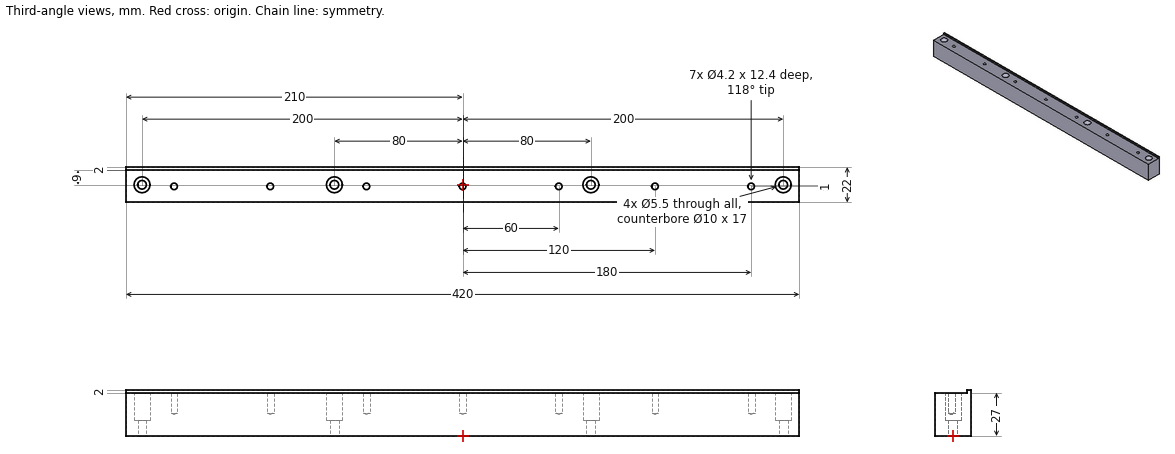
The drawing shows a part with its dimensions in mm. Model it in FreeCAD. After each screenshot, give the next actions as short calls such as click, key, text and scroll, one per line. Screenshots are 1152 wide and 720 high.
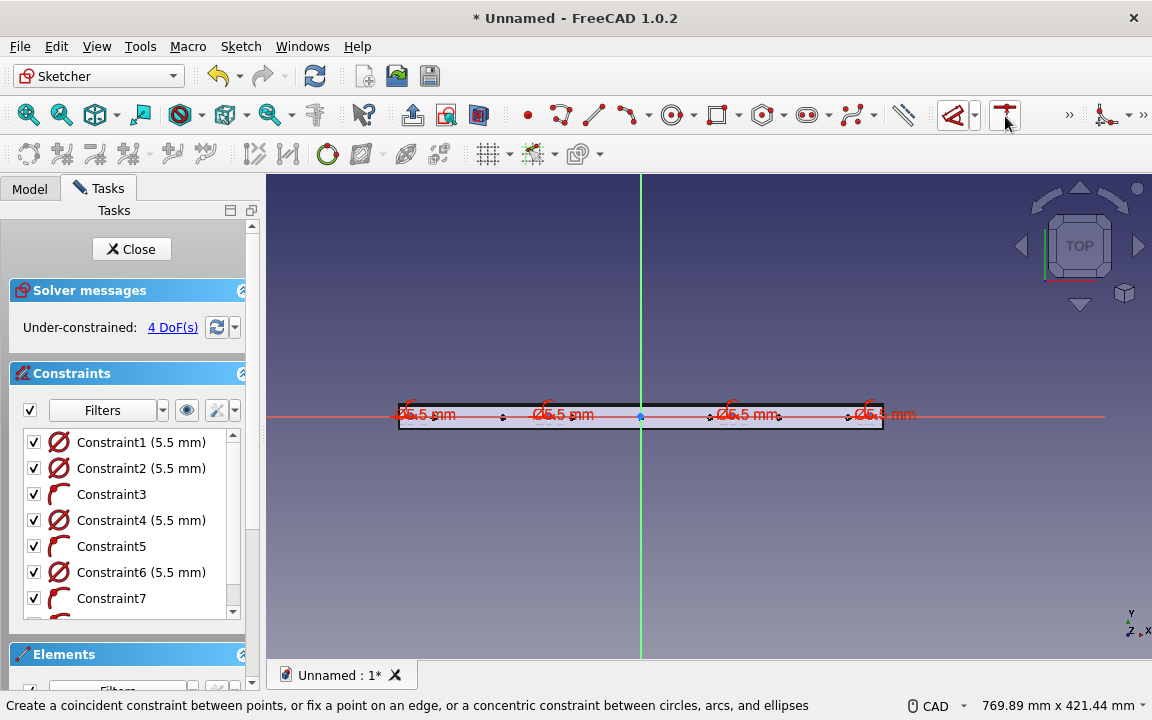
click(733, 417)
click(687, 451)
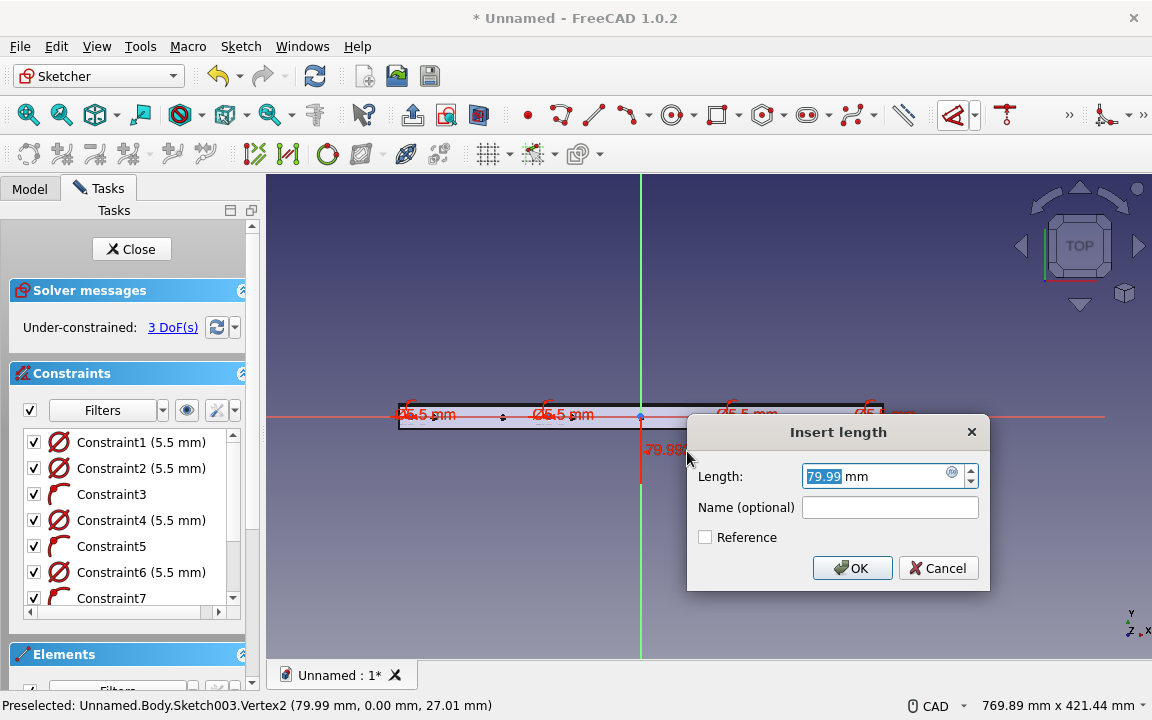
text(80)
key(Return)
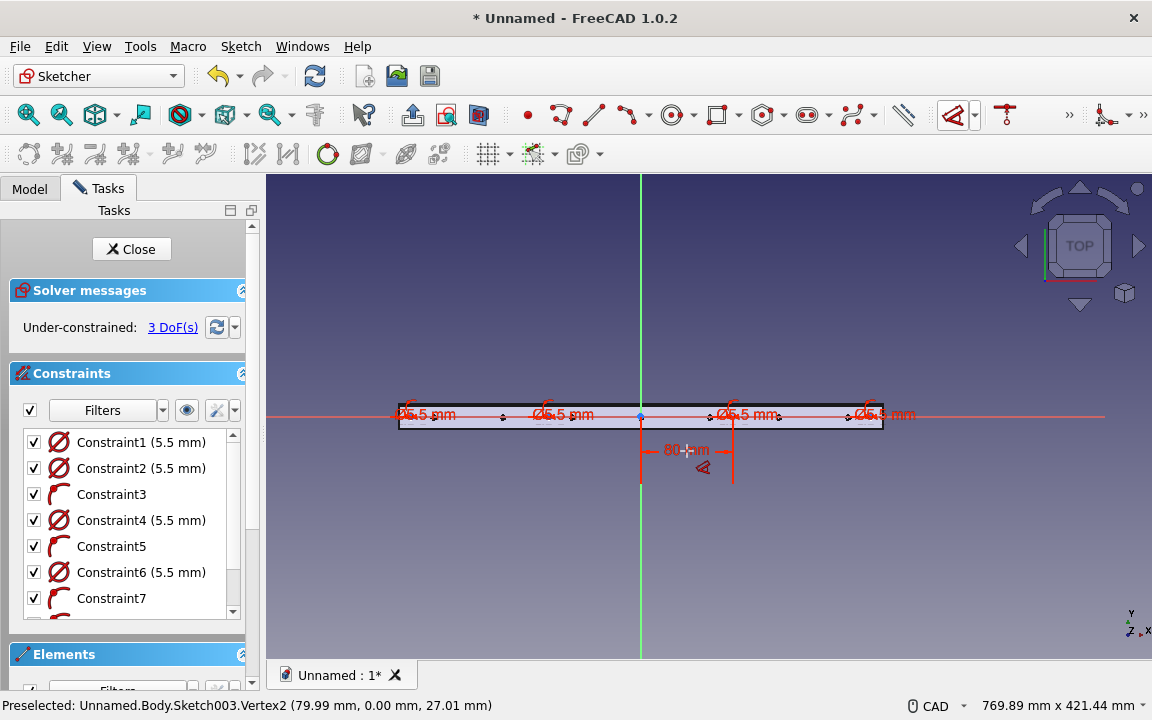
click(549, 417)
click(595, 451)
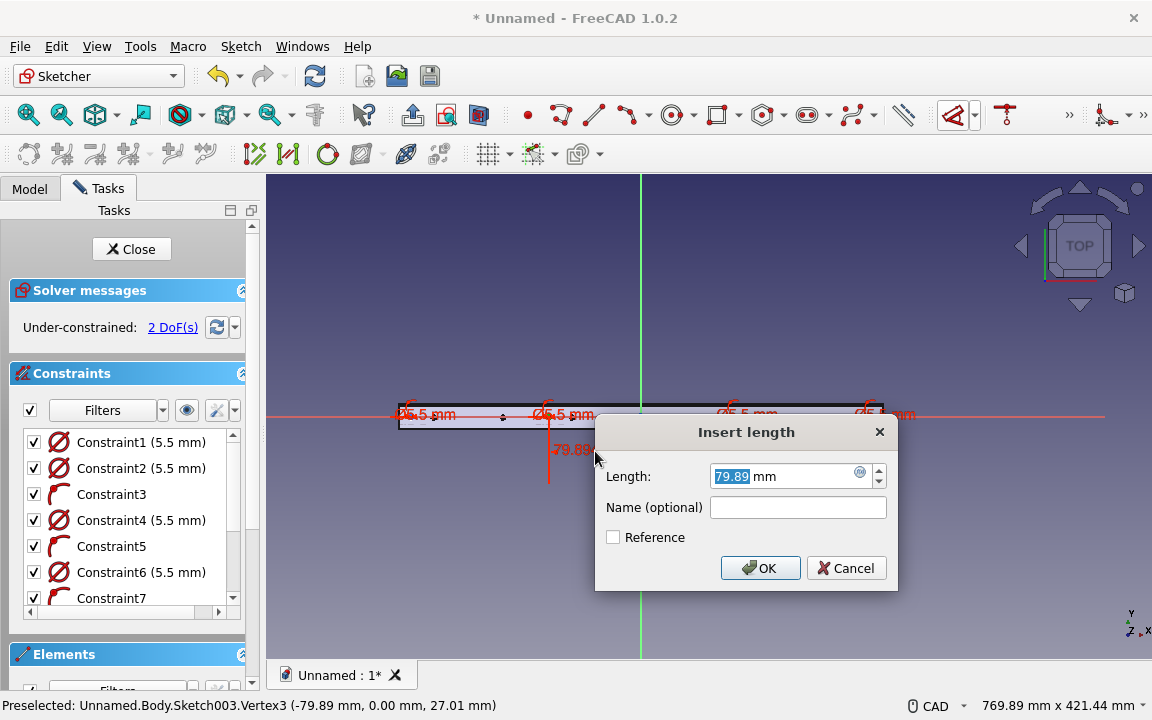
text(80)
key(Return)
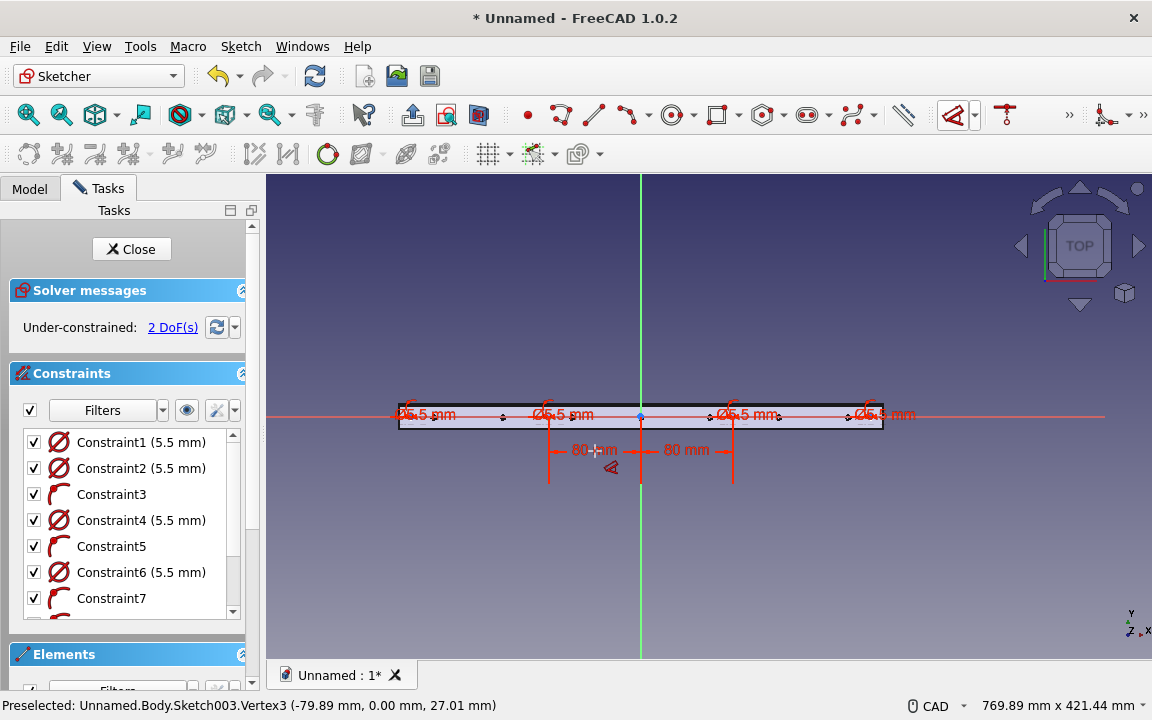
click(871, 417)
click(809, 451)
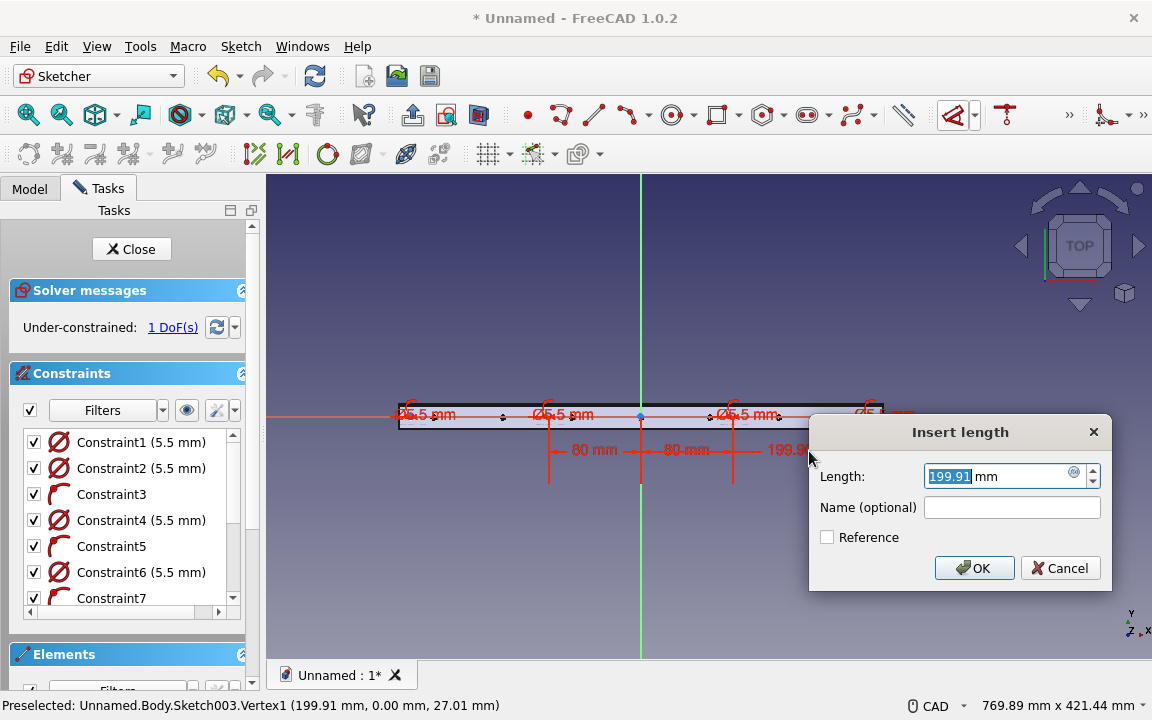
text(200)
key(Return)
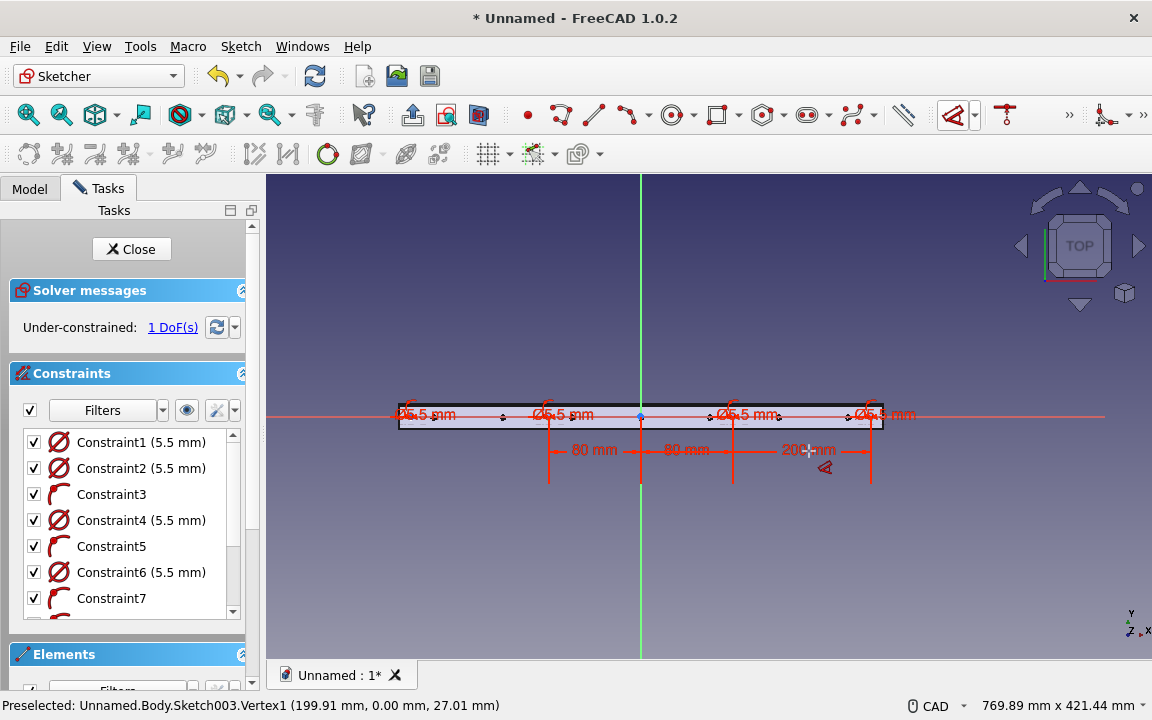
click(411, 417)
click(473, 451)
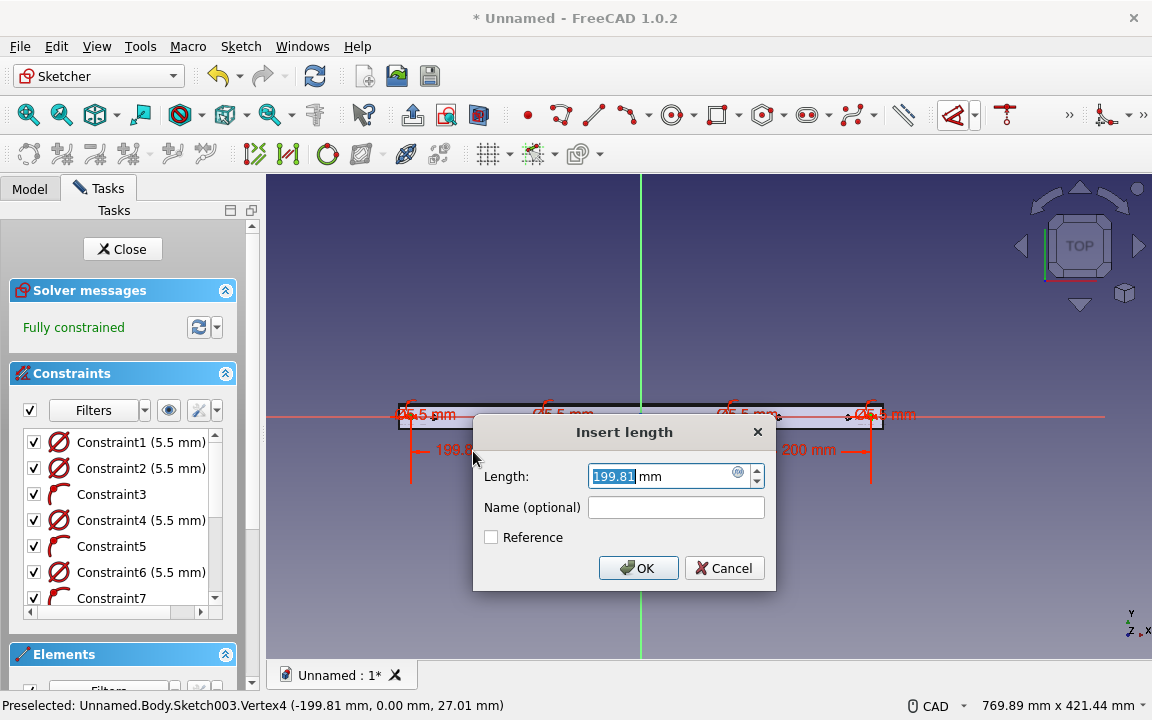
text(200)
key(Return)
key(Escape)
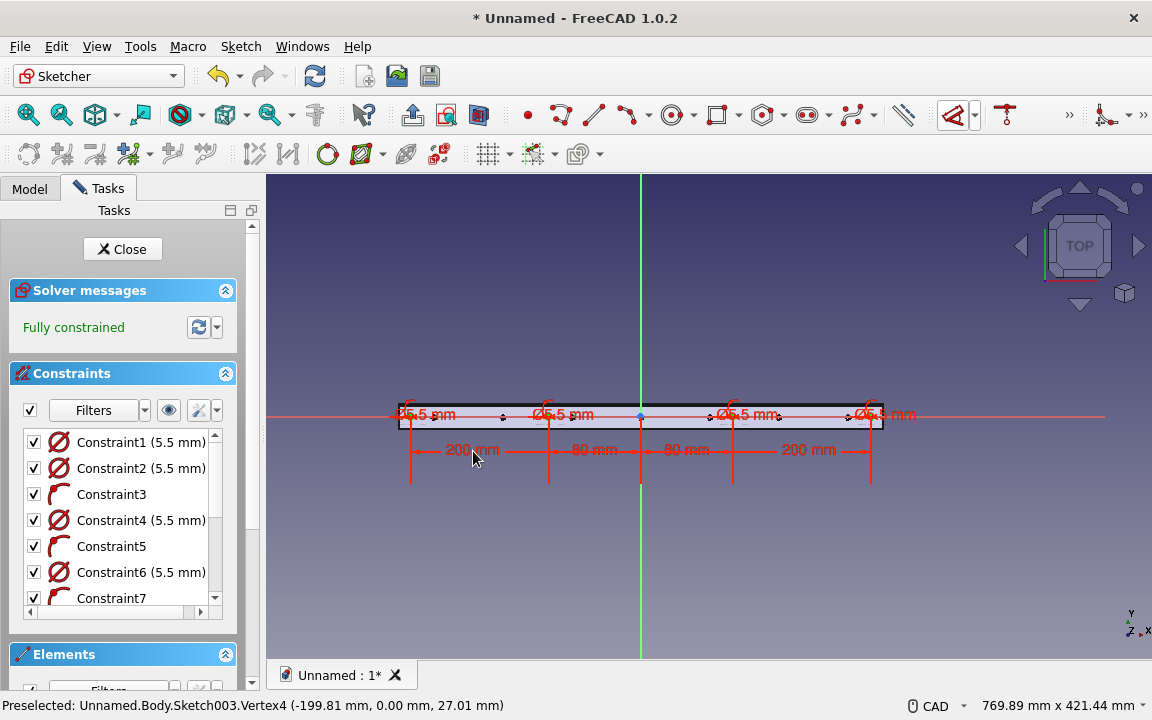
click(123, 249)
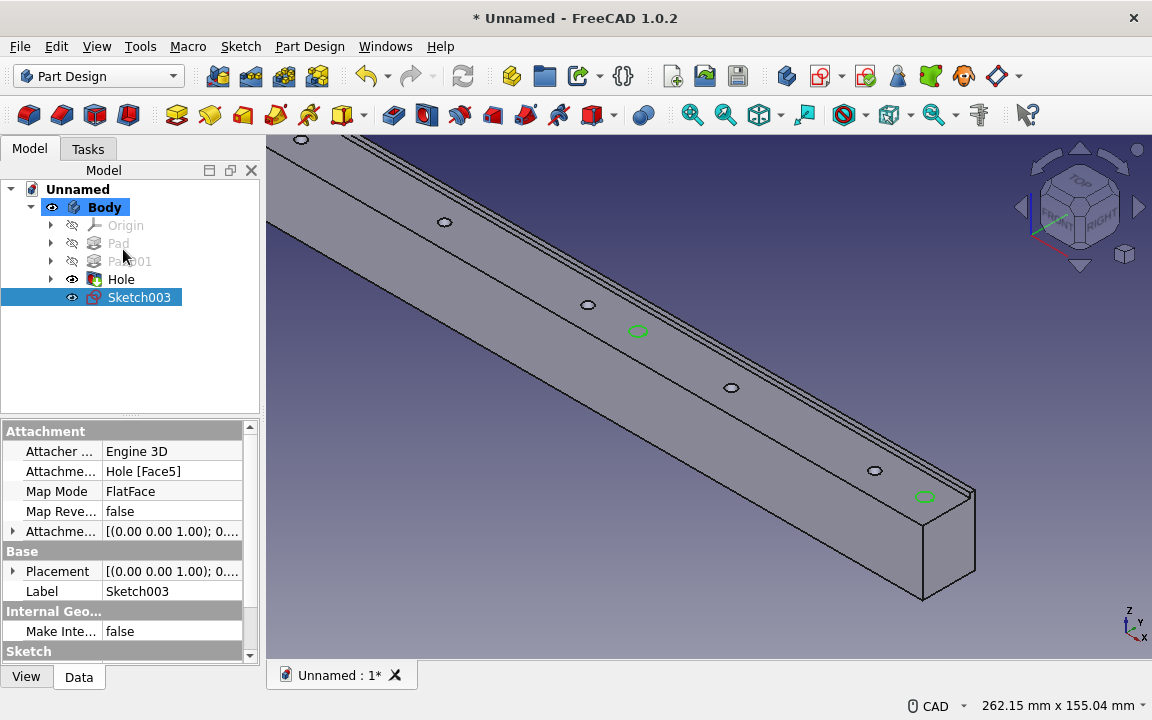
click(427, 116)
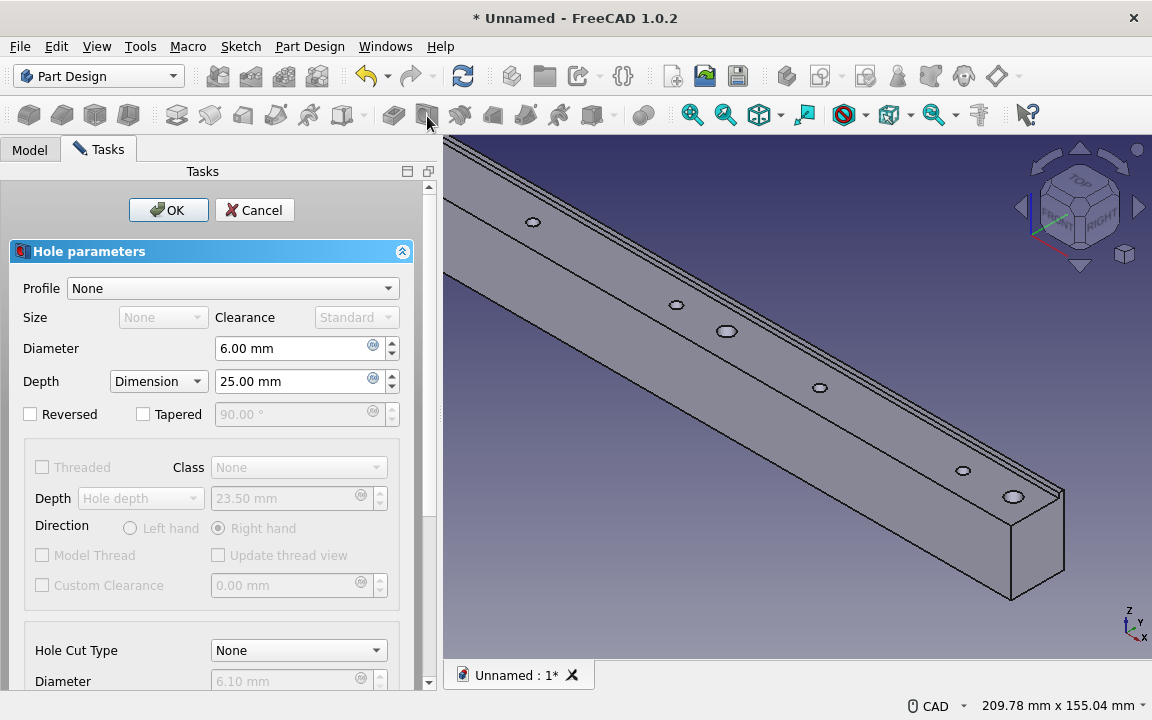
triple_click(300, 348)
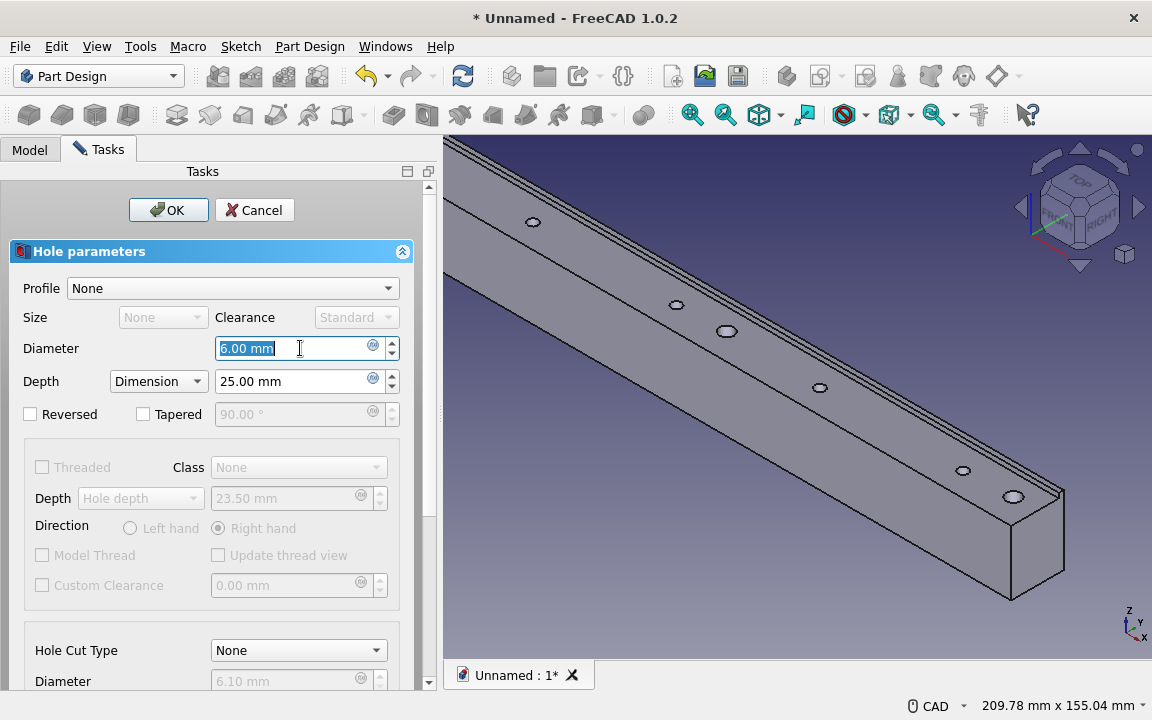
text(5.5)
key(Tab)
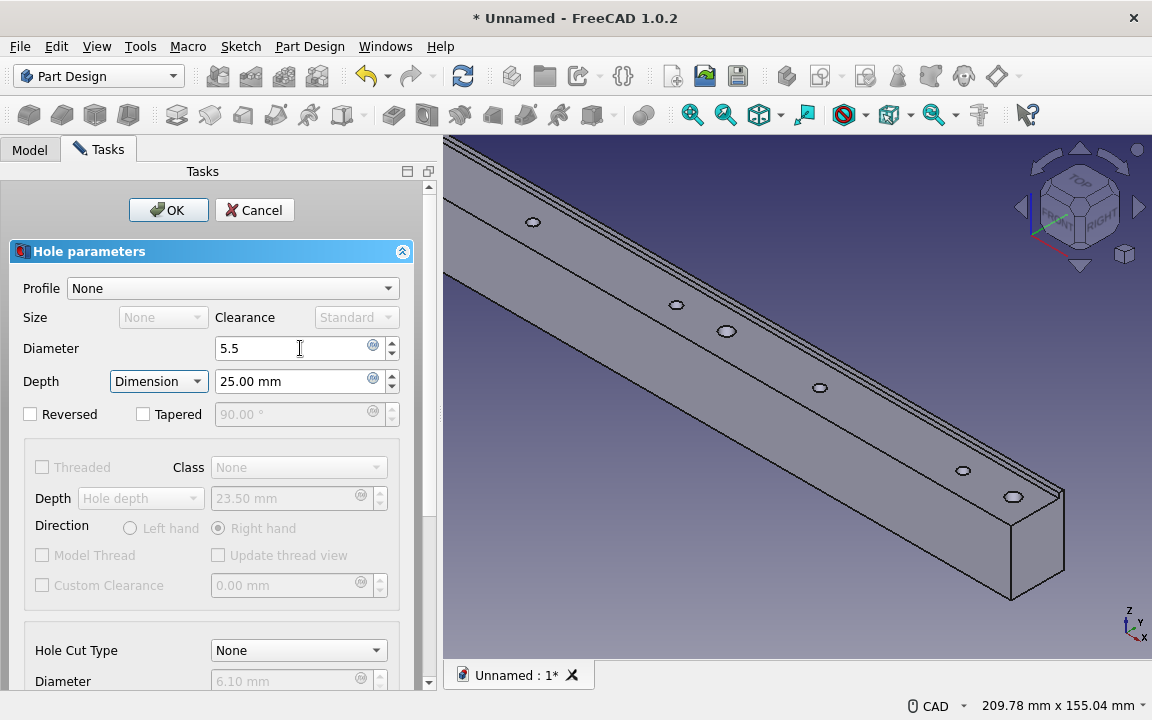
click(160, 382)